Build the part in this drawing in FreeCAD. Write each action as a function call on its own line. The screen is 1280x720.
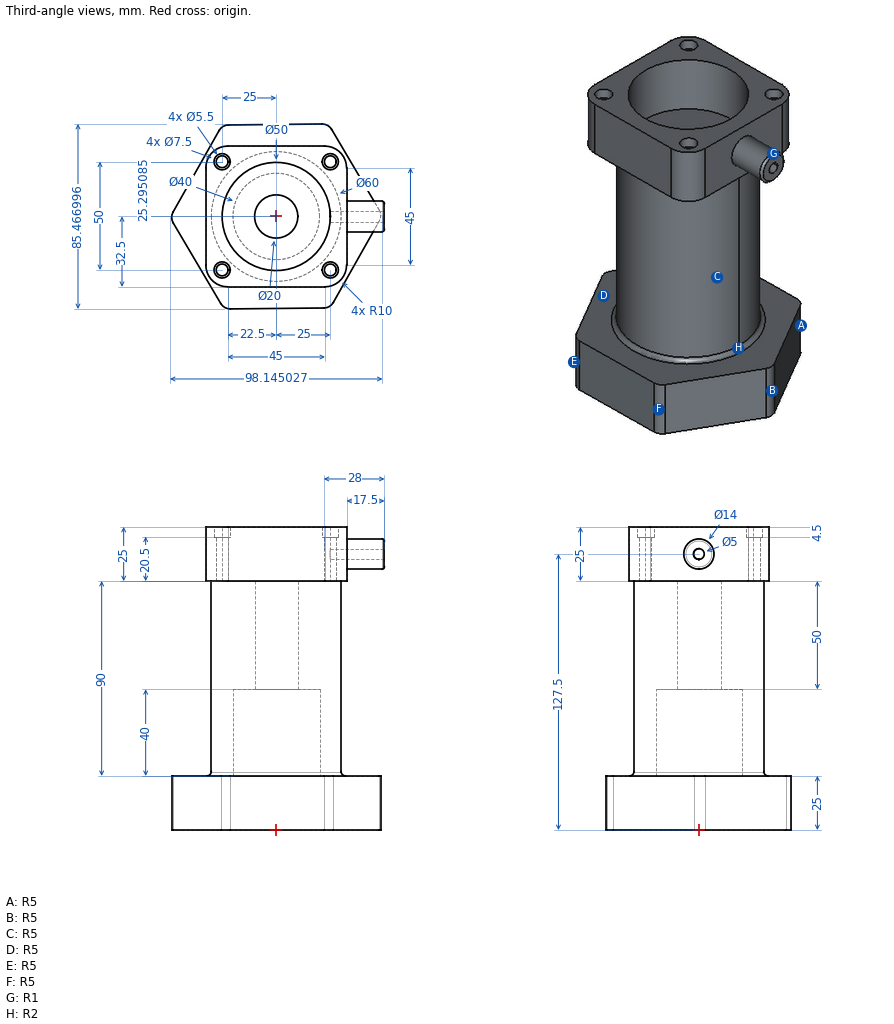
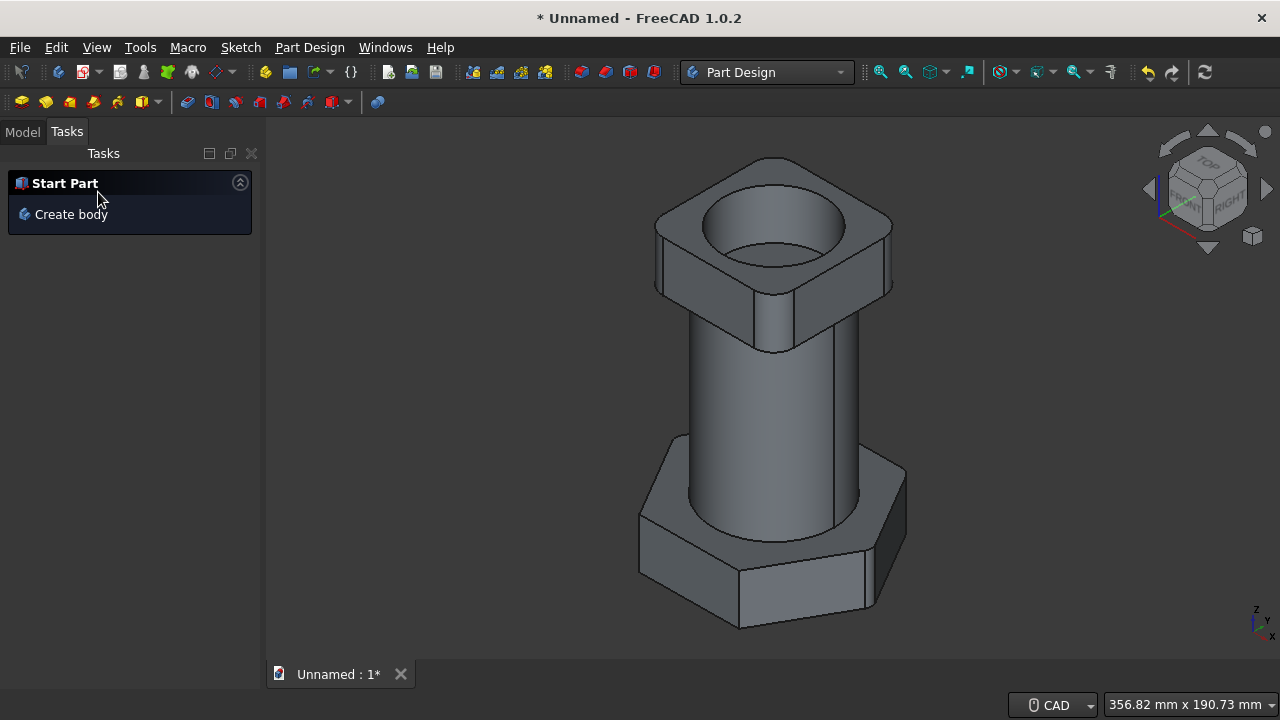
key(2)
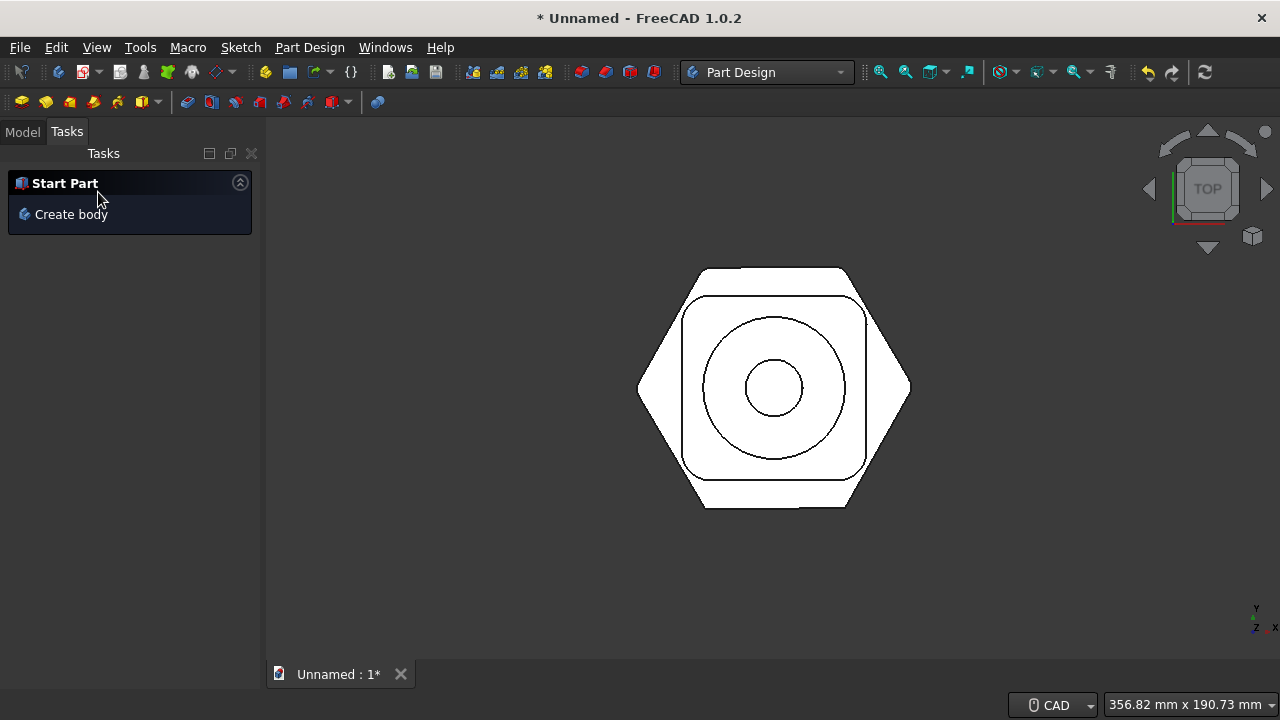
click(882, 72)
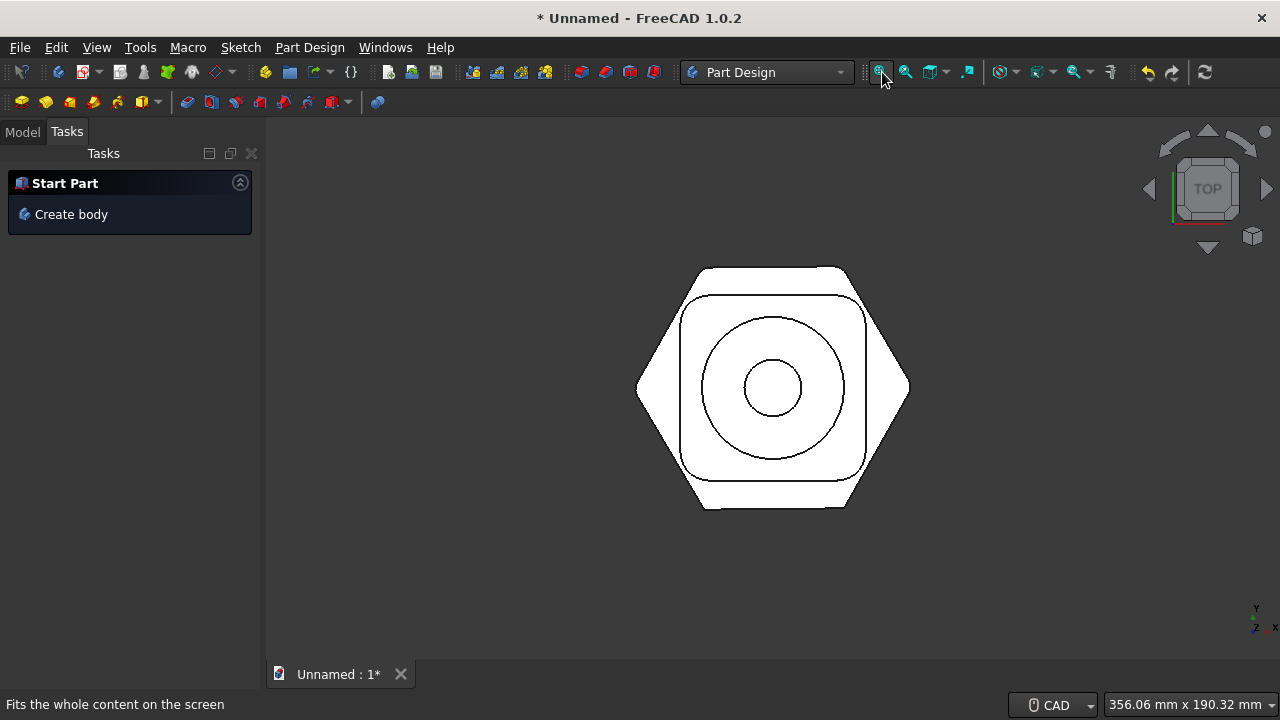
key(1)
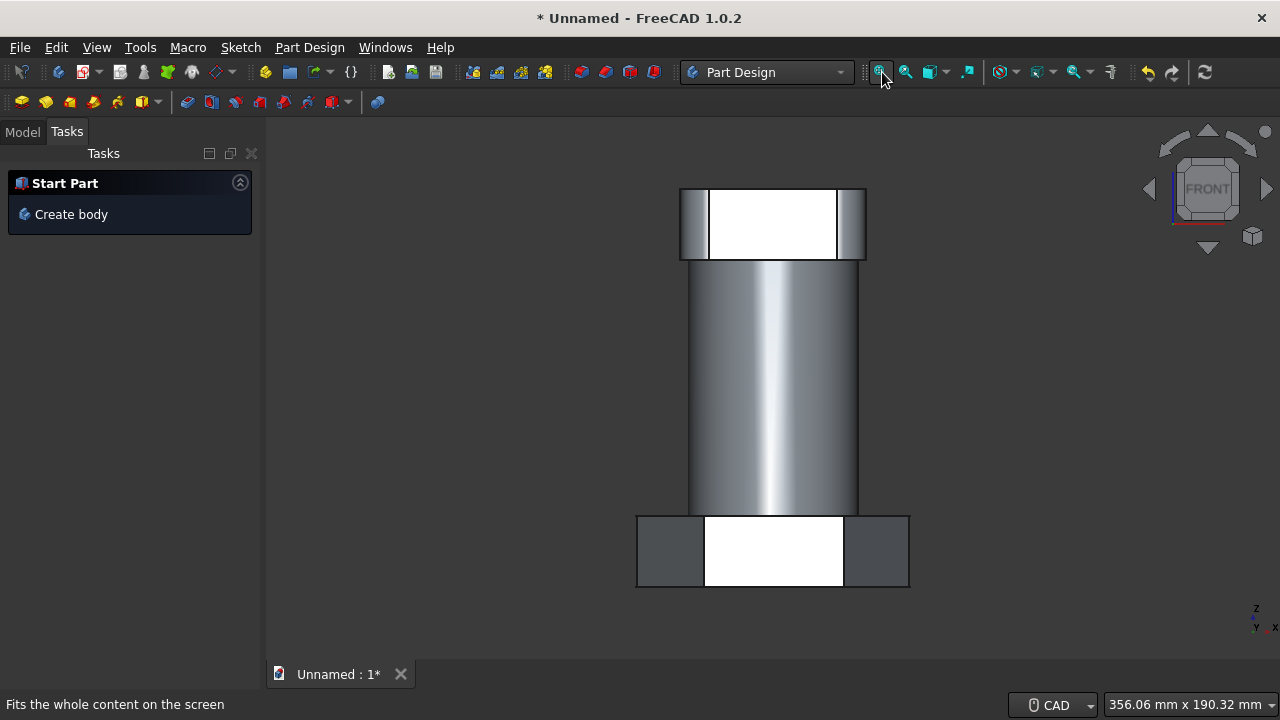
click(704, 551)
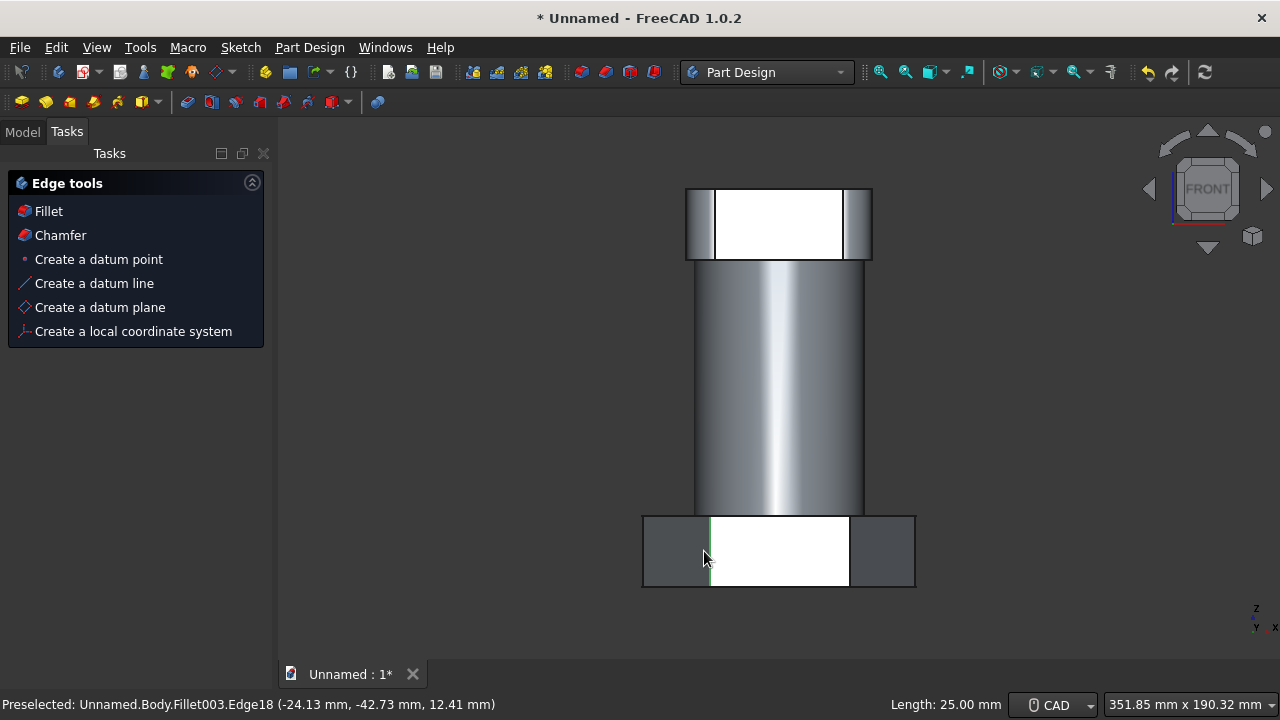
click(582, 72)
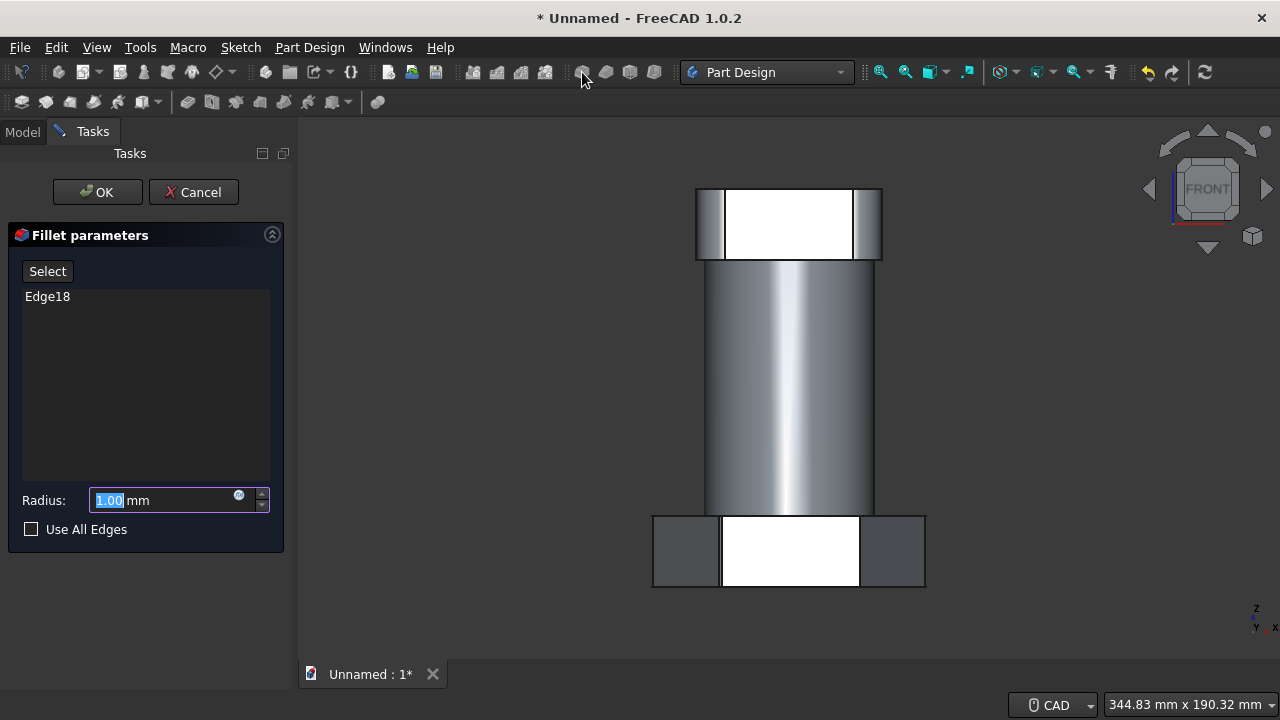
text(5)
key(Tab)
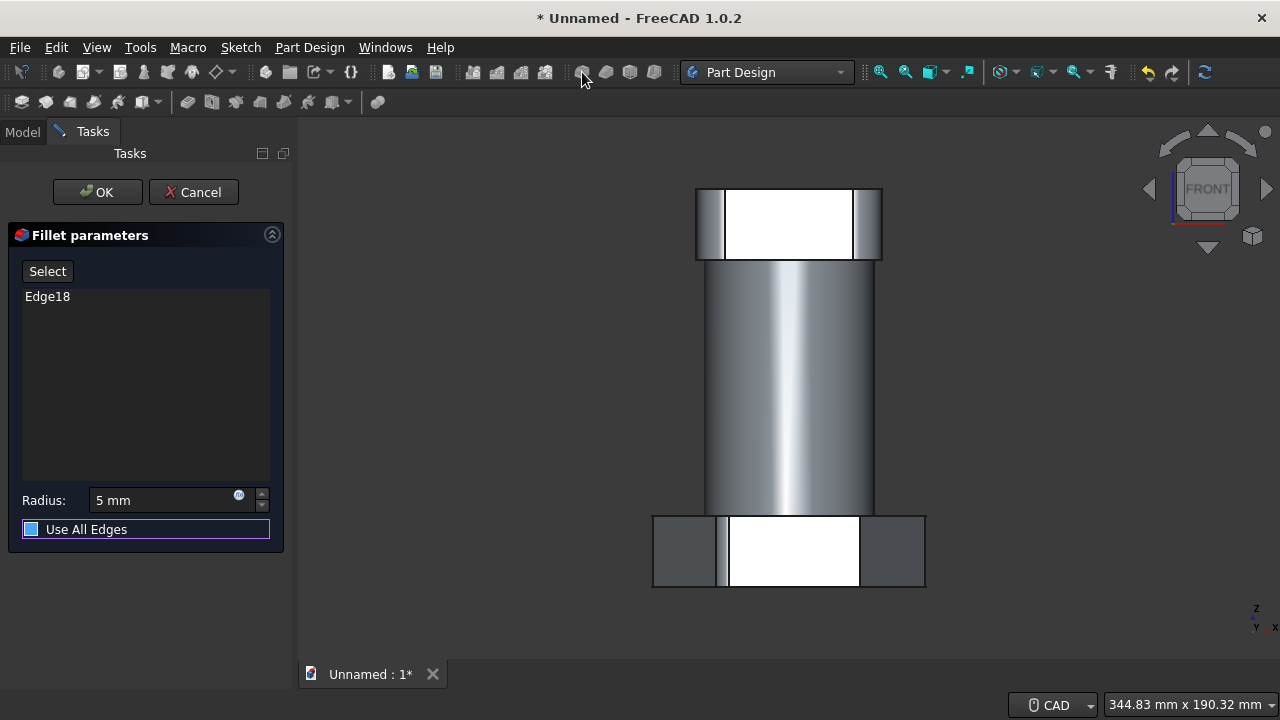
click(98, 192)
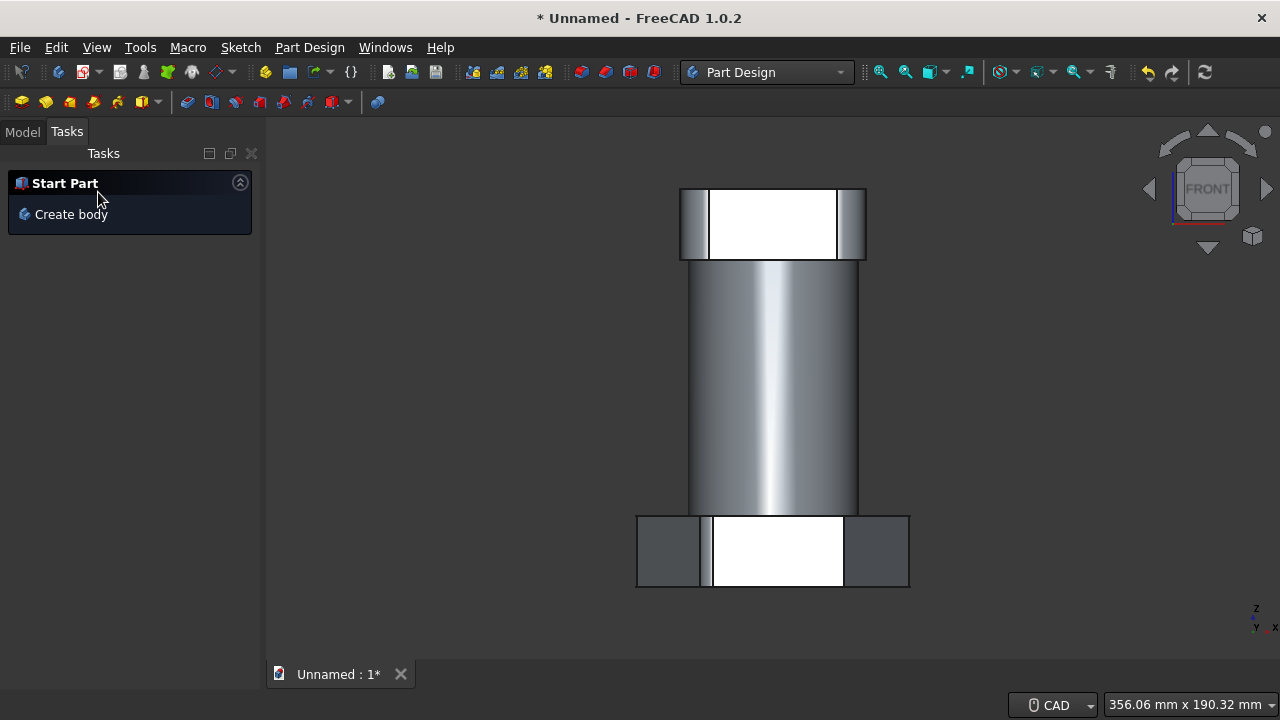
key(0)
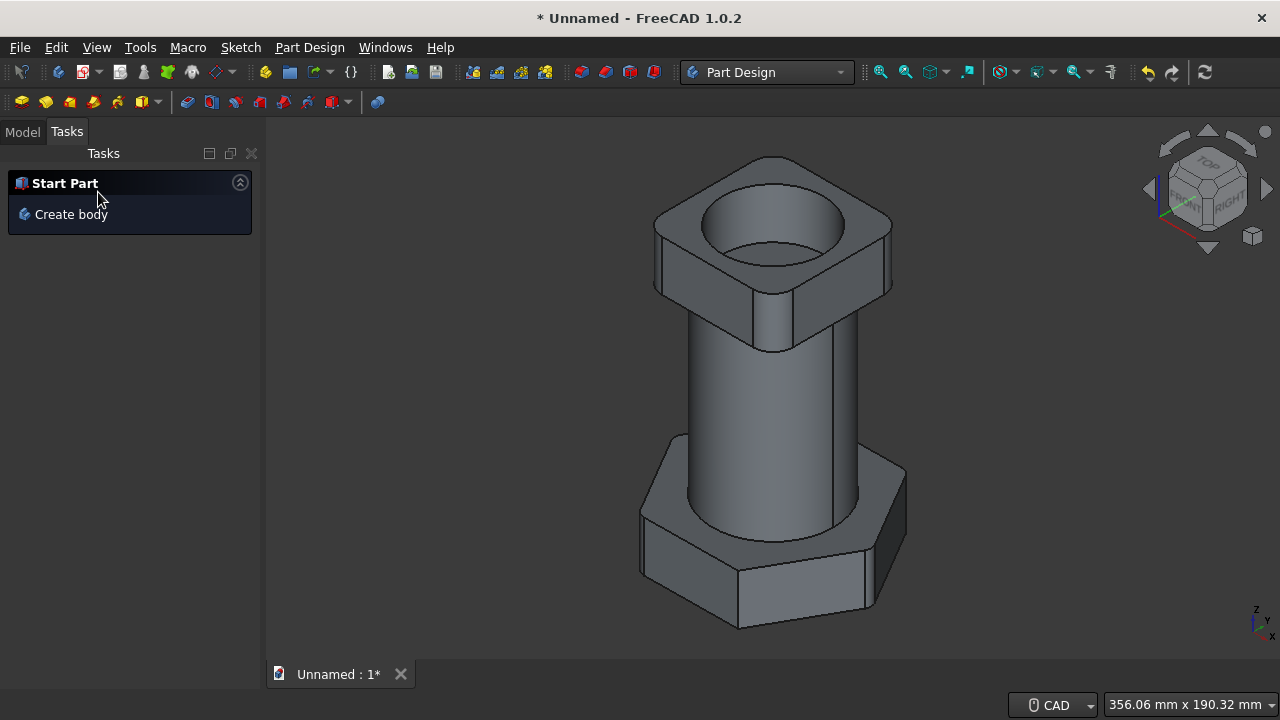
click(738, 599)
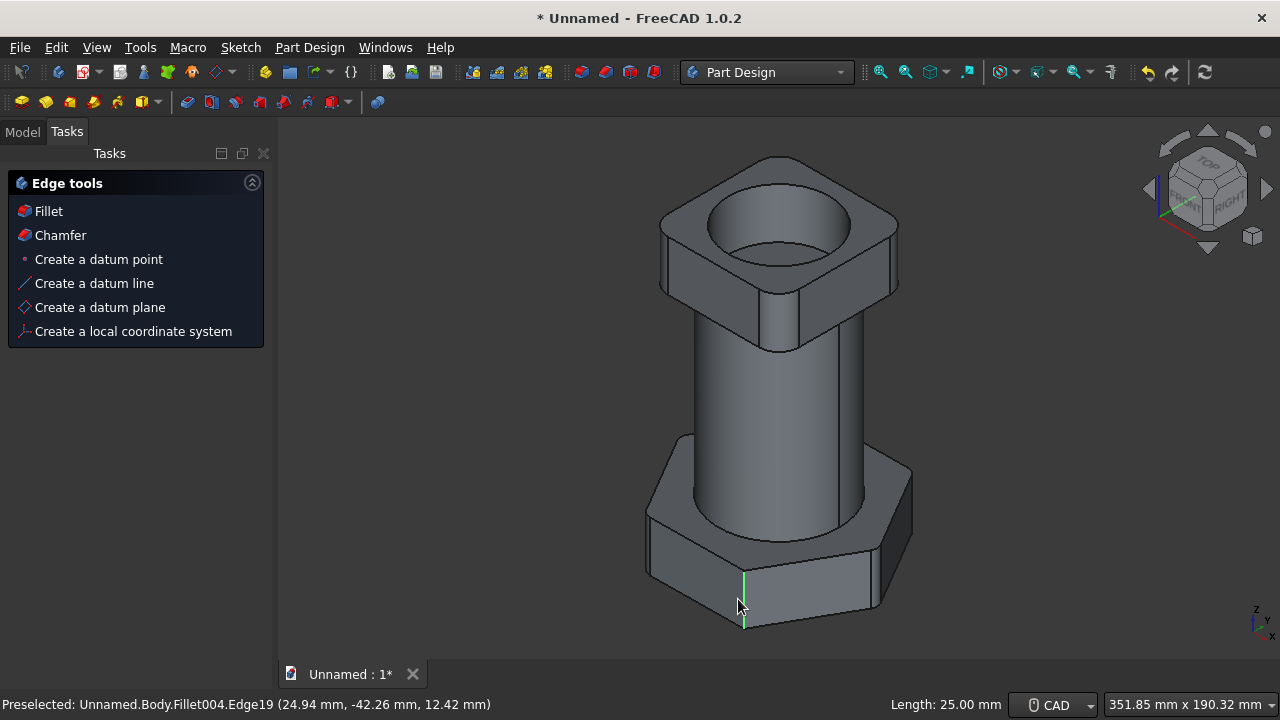
click(582, 72)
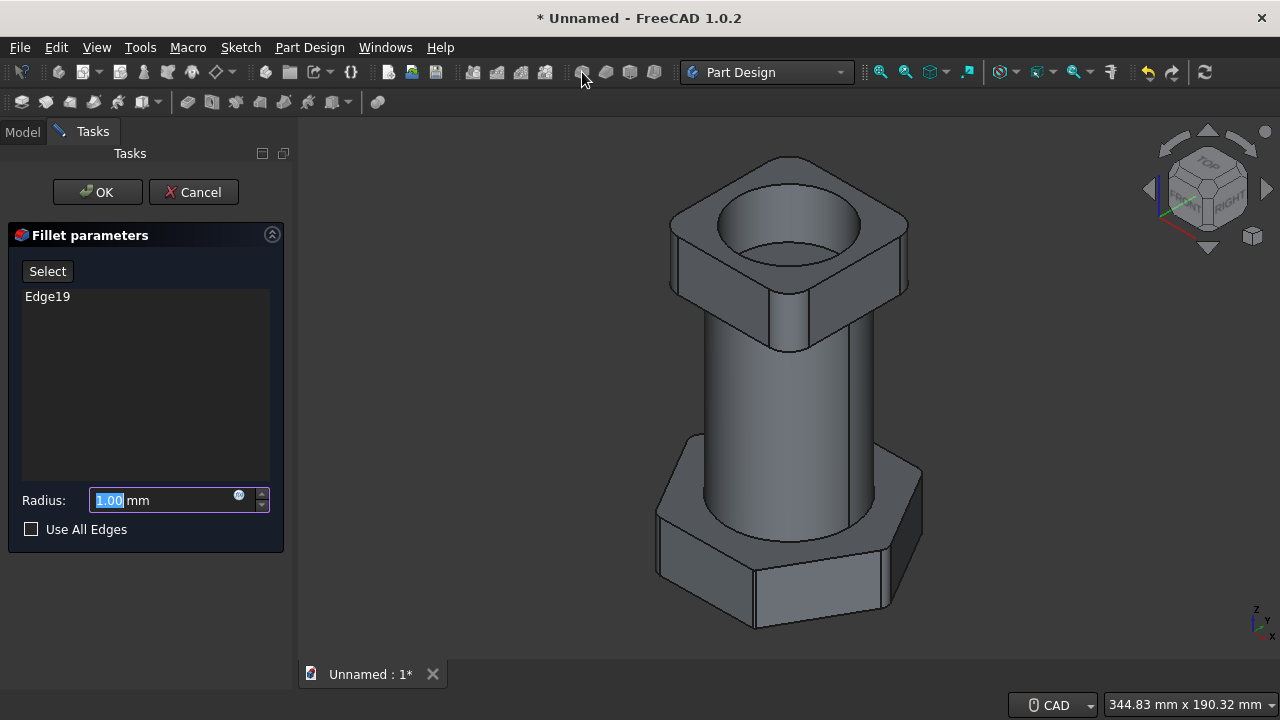
text(5)
key(Tab)